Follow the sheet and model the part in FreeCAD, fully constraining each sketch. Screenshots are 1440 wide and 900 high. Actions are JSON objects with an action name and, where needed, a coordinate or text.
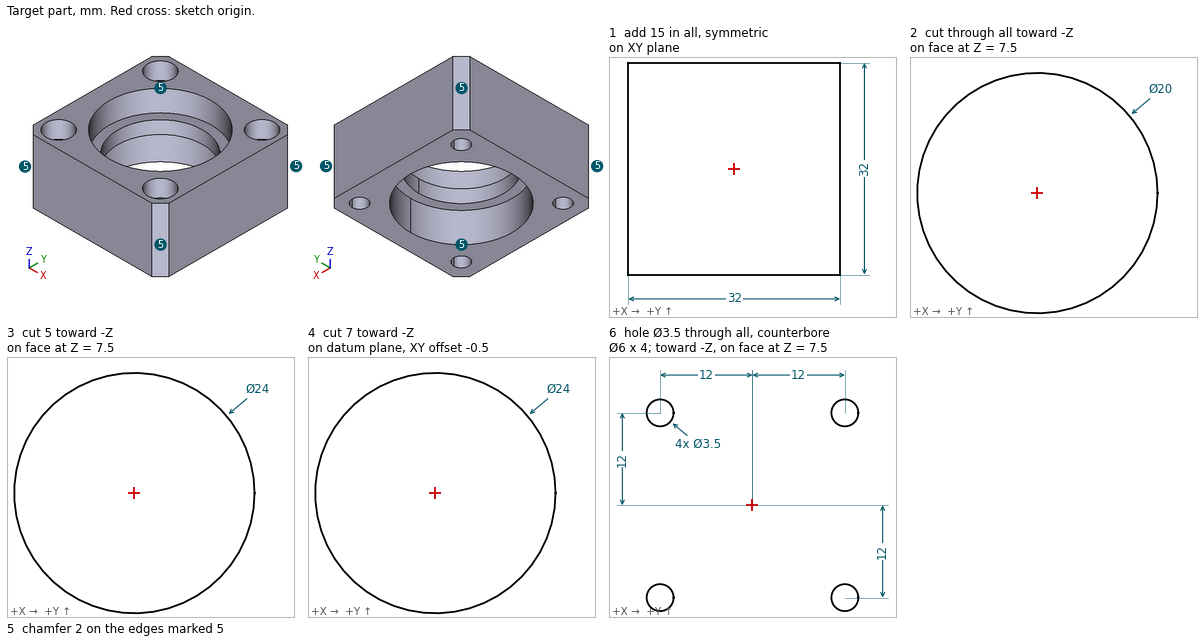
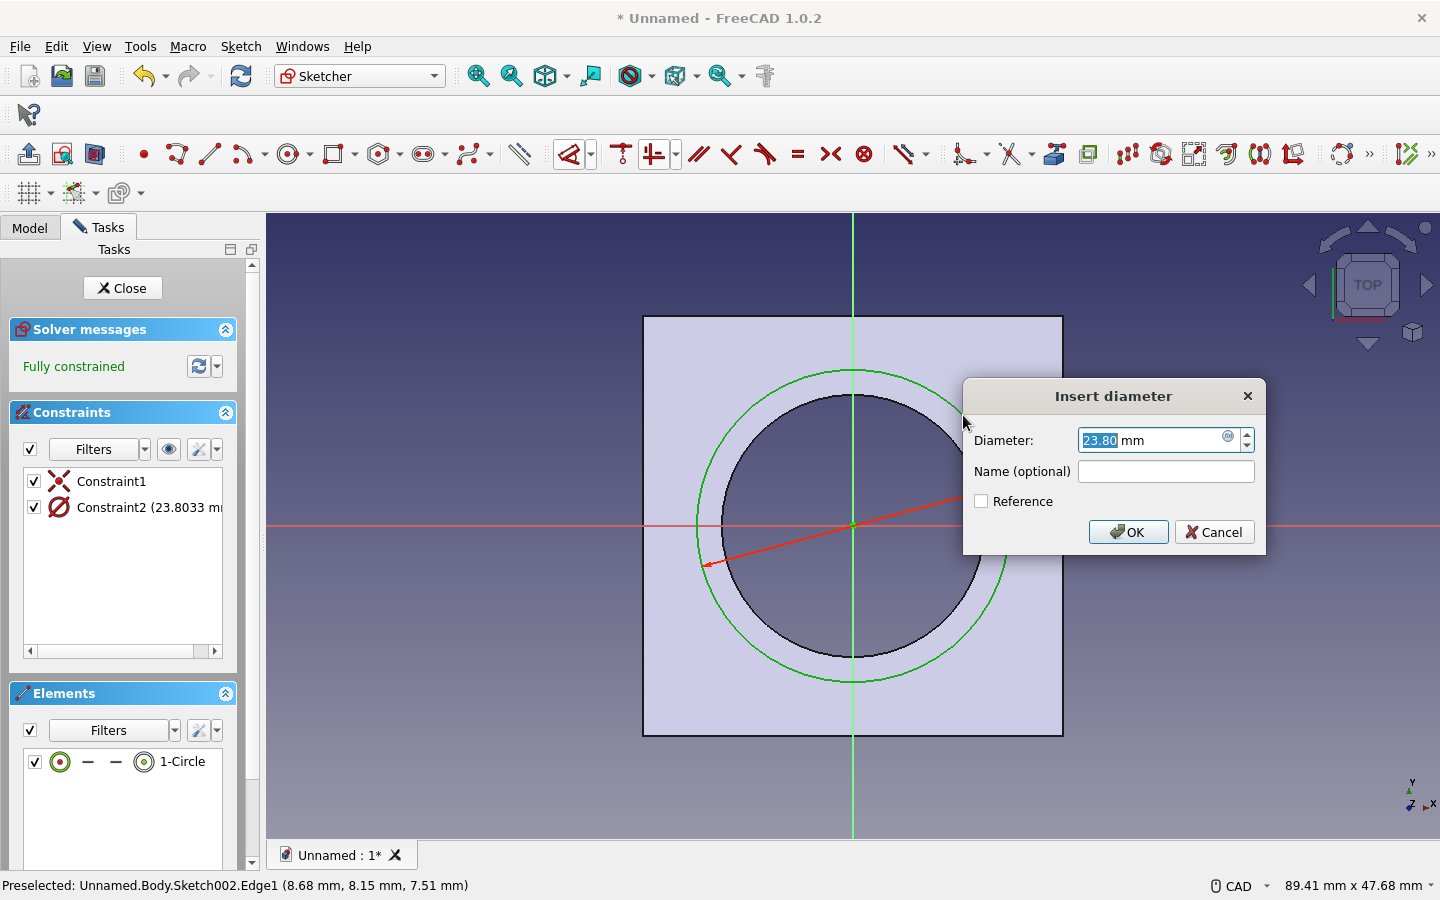
{"action": "type", "text": "24"}
{"action": "key", "text": "Return"}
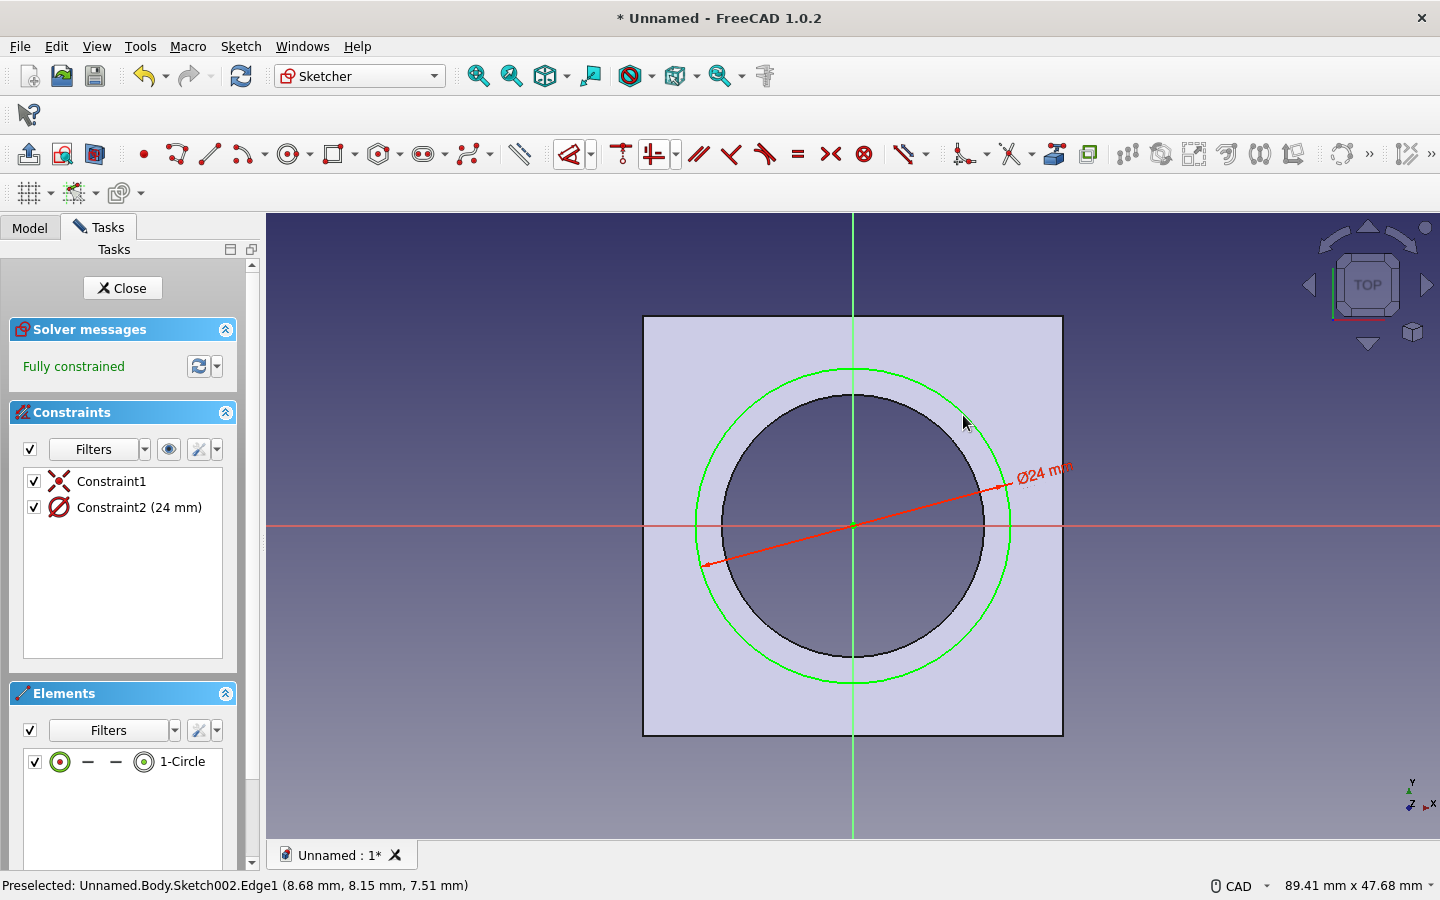
{"action": "left_click", "coordinate": [123, 288]}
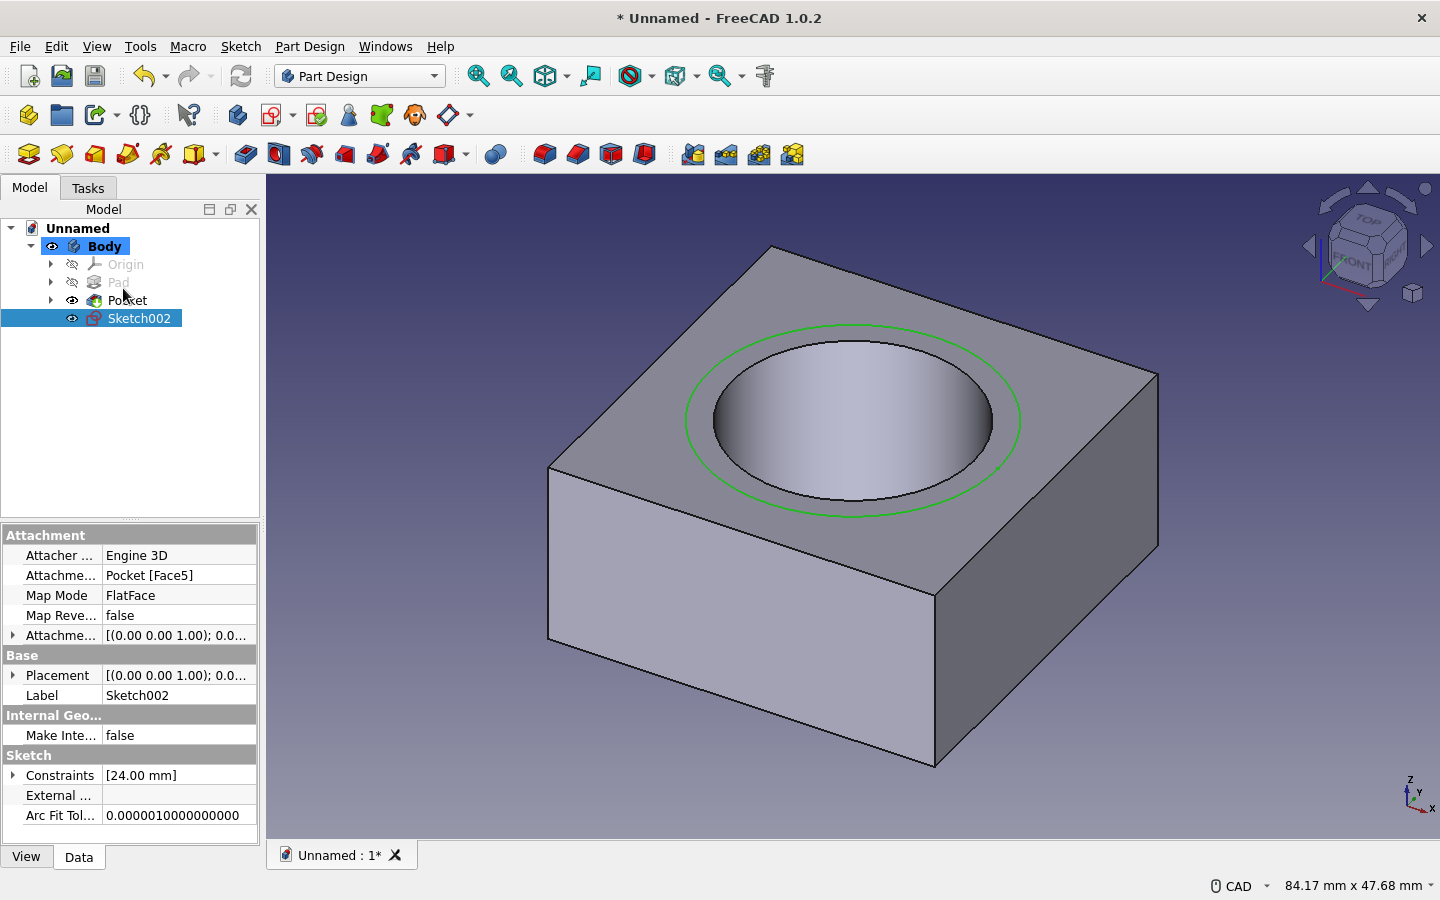
{"action": "left_click", "coordinate": [246, 154]}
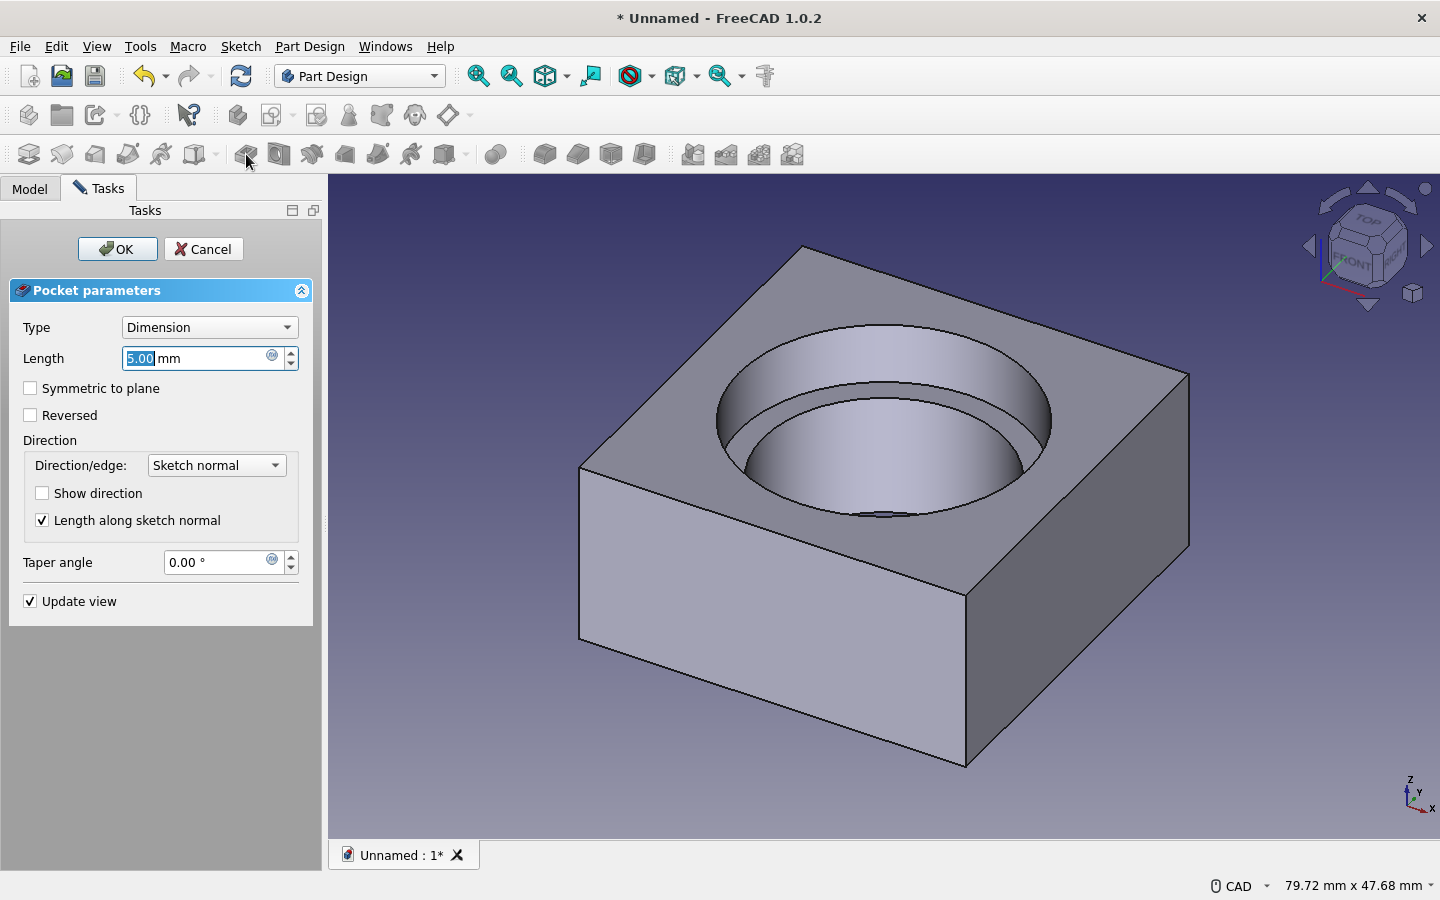
{"action": "type", "text": "5"}
{"action": "key", "text": "Tab"}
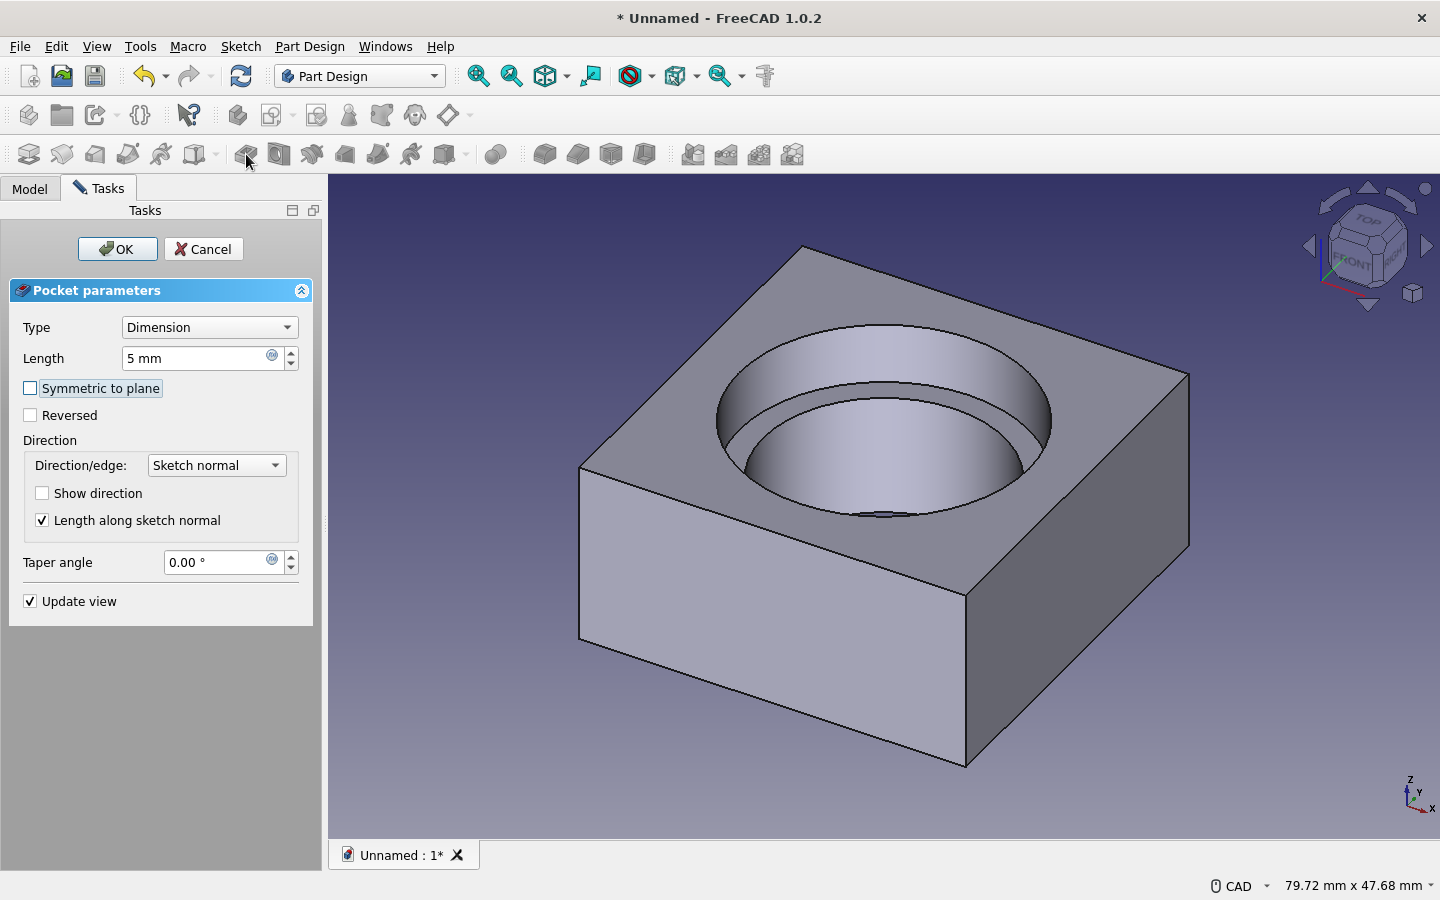
{"action": "left_click", "coordinate": [118, 249]}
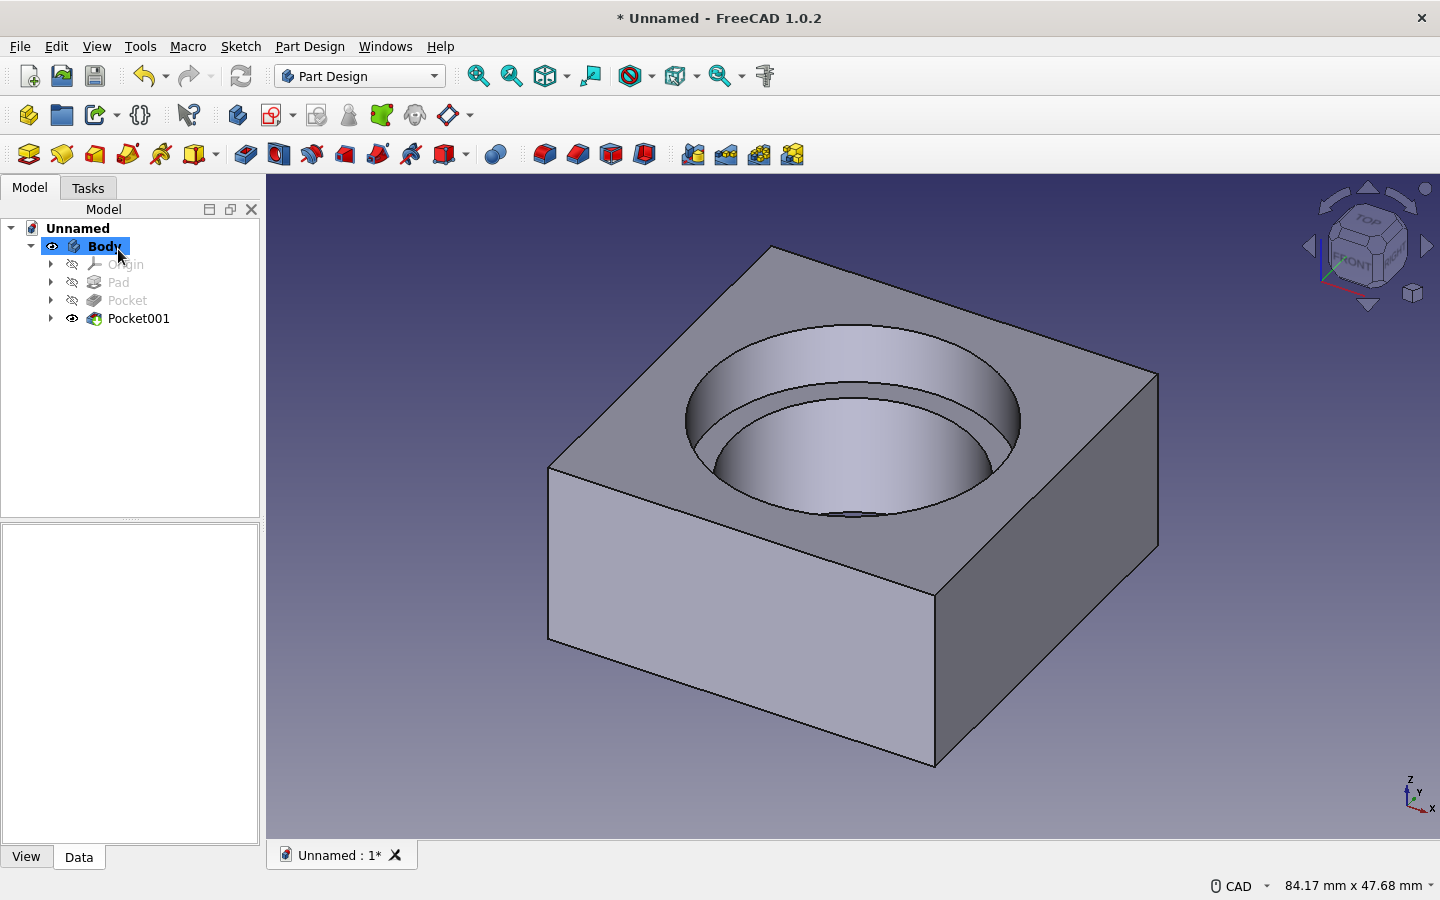
{"action": "left_click", "coordinate": [51, 264]}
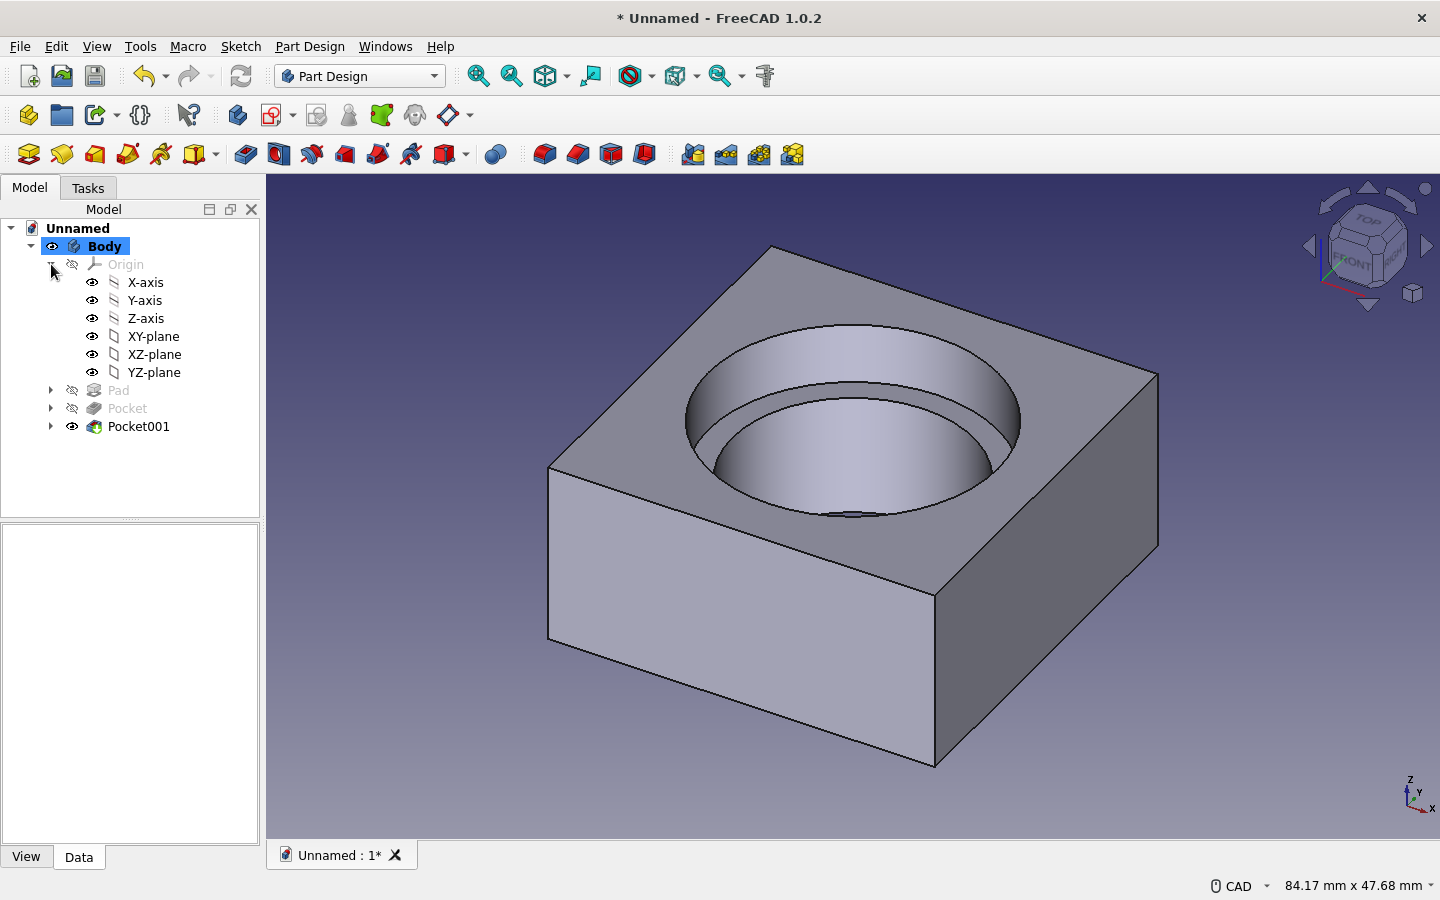
{"action": "left_click", "coordinate": [137, 336]}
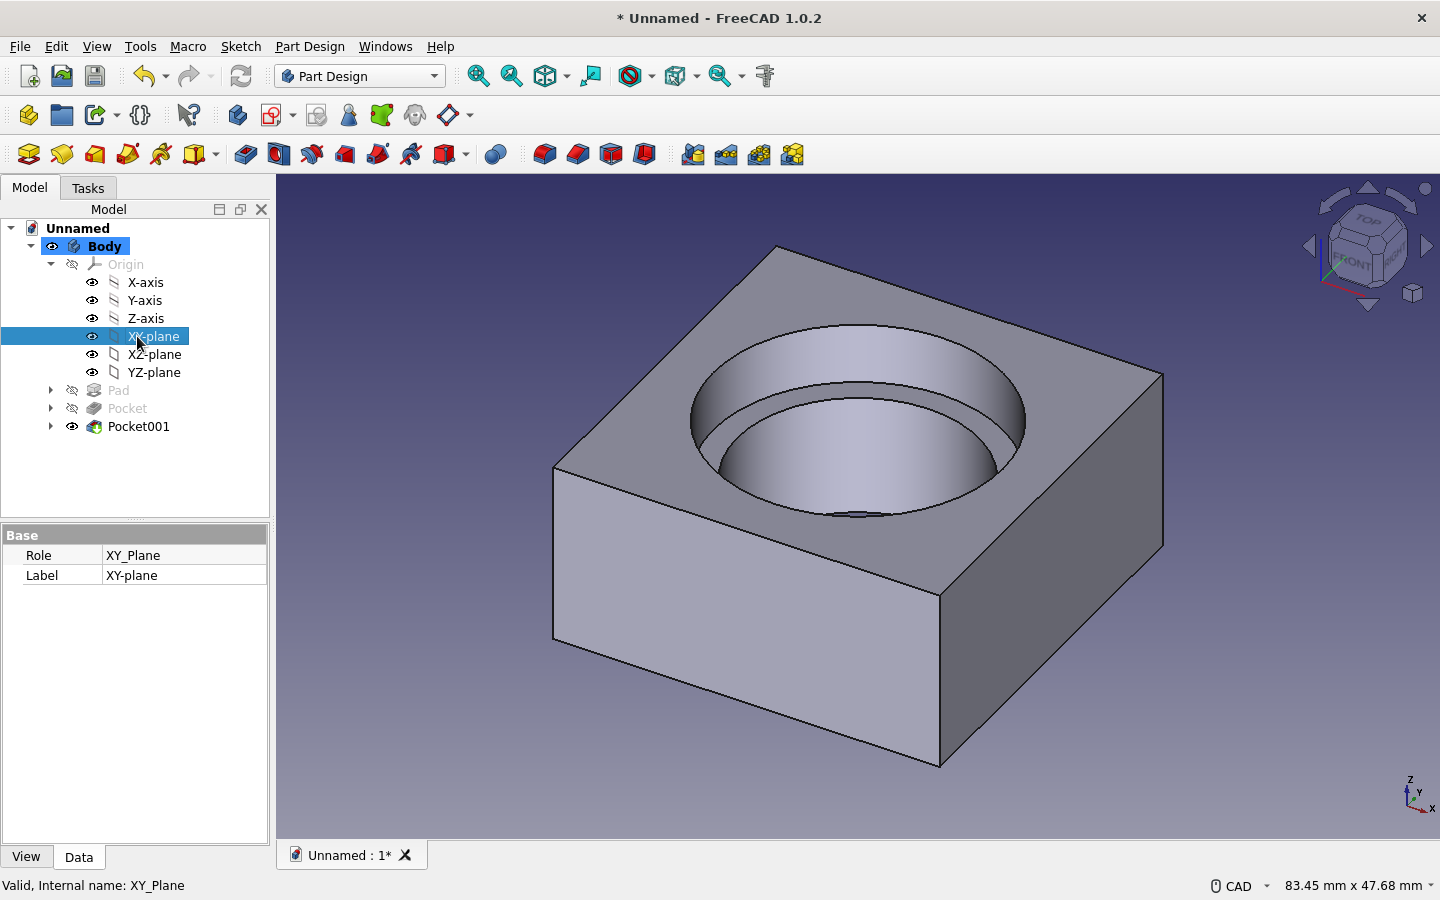
{"action": "left_click", "coordinate": [448, 116]}